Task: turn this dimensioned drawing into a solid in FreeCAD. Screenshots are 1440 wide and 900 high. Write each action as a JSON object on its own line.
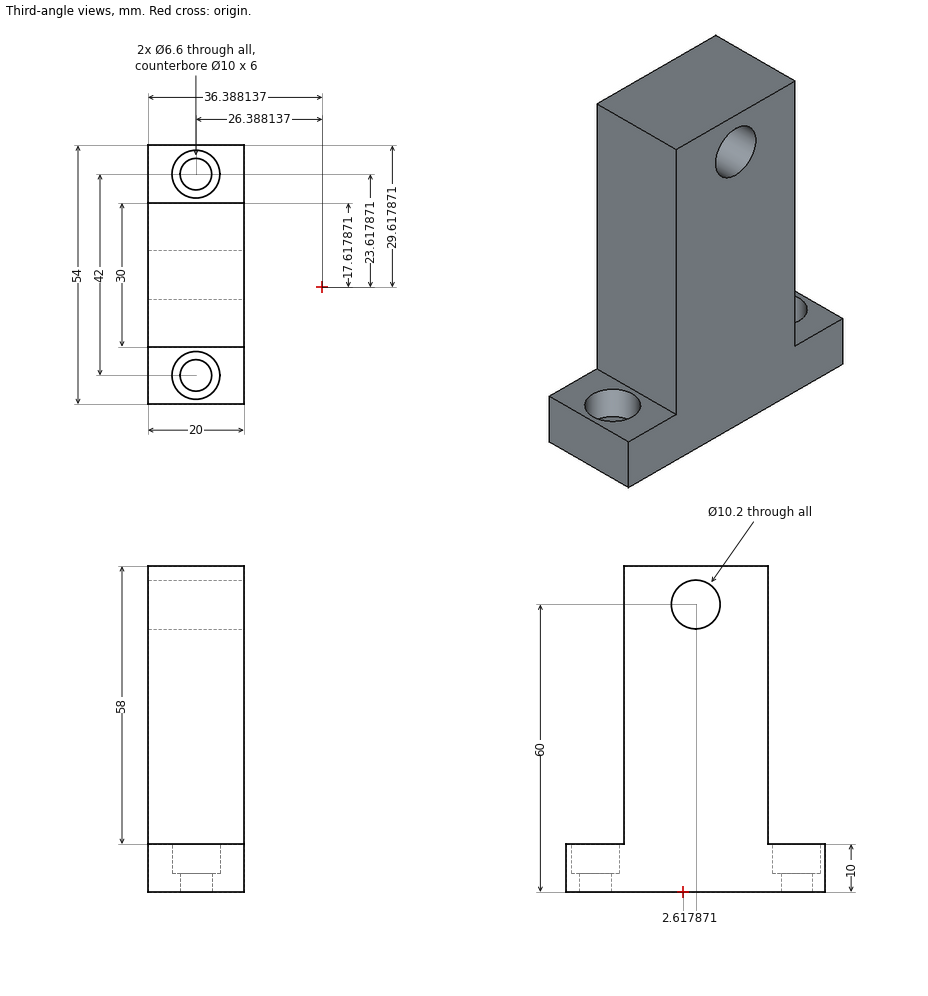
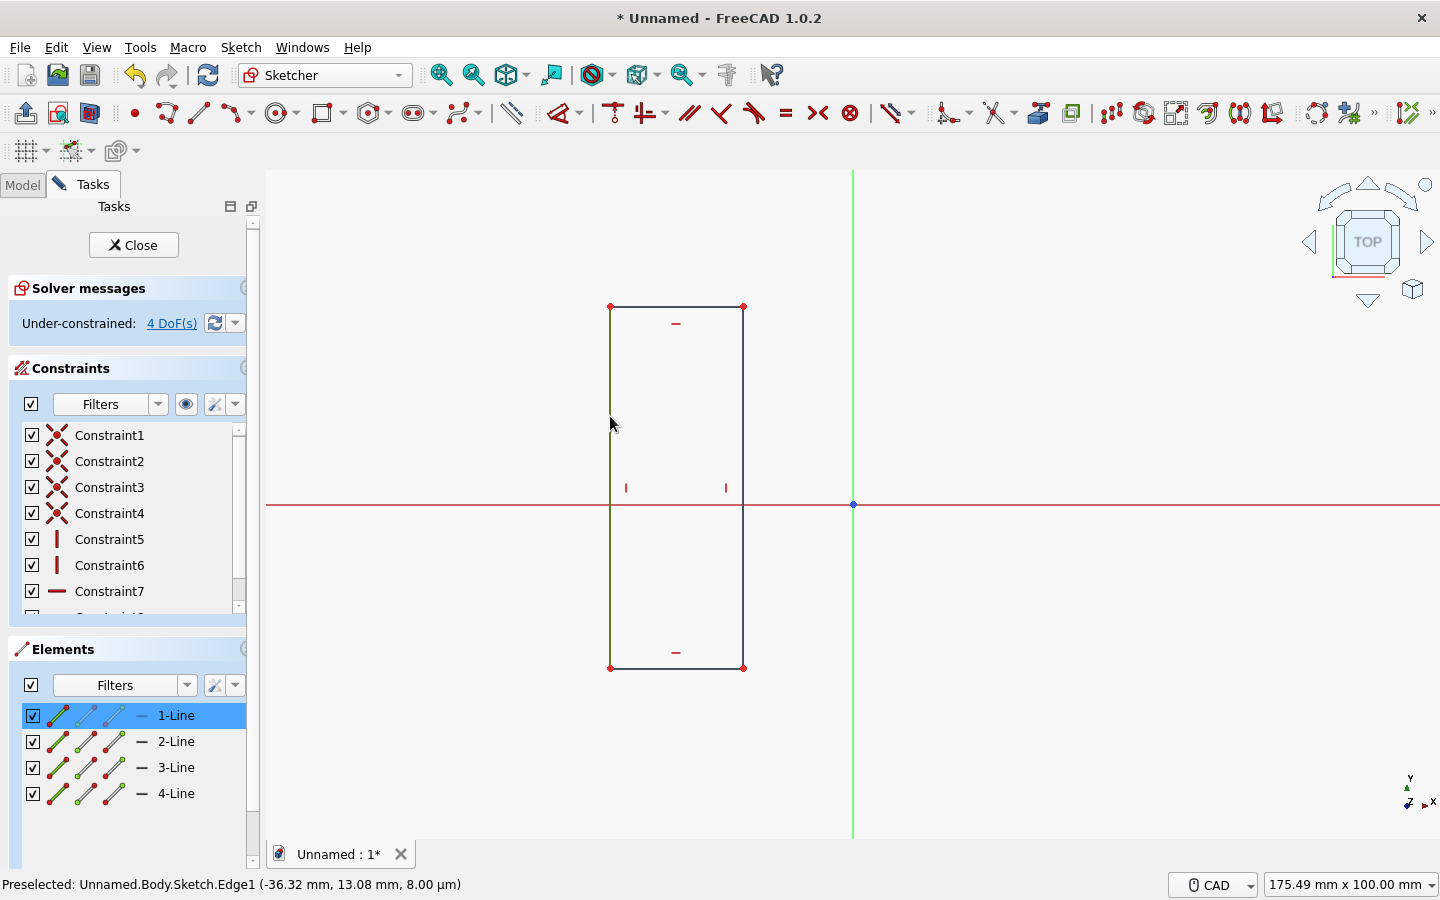
{"action": "left_click", "coordinate": [582, 114]}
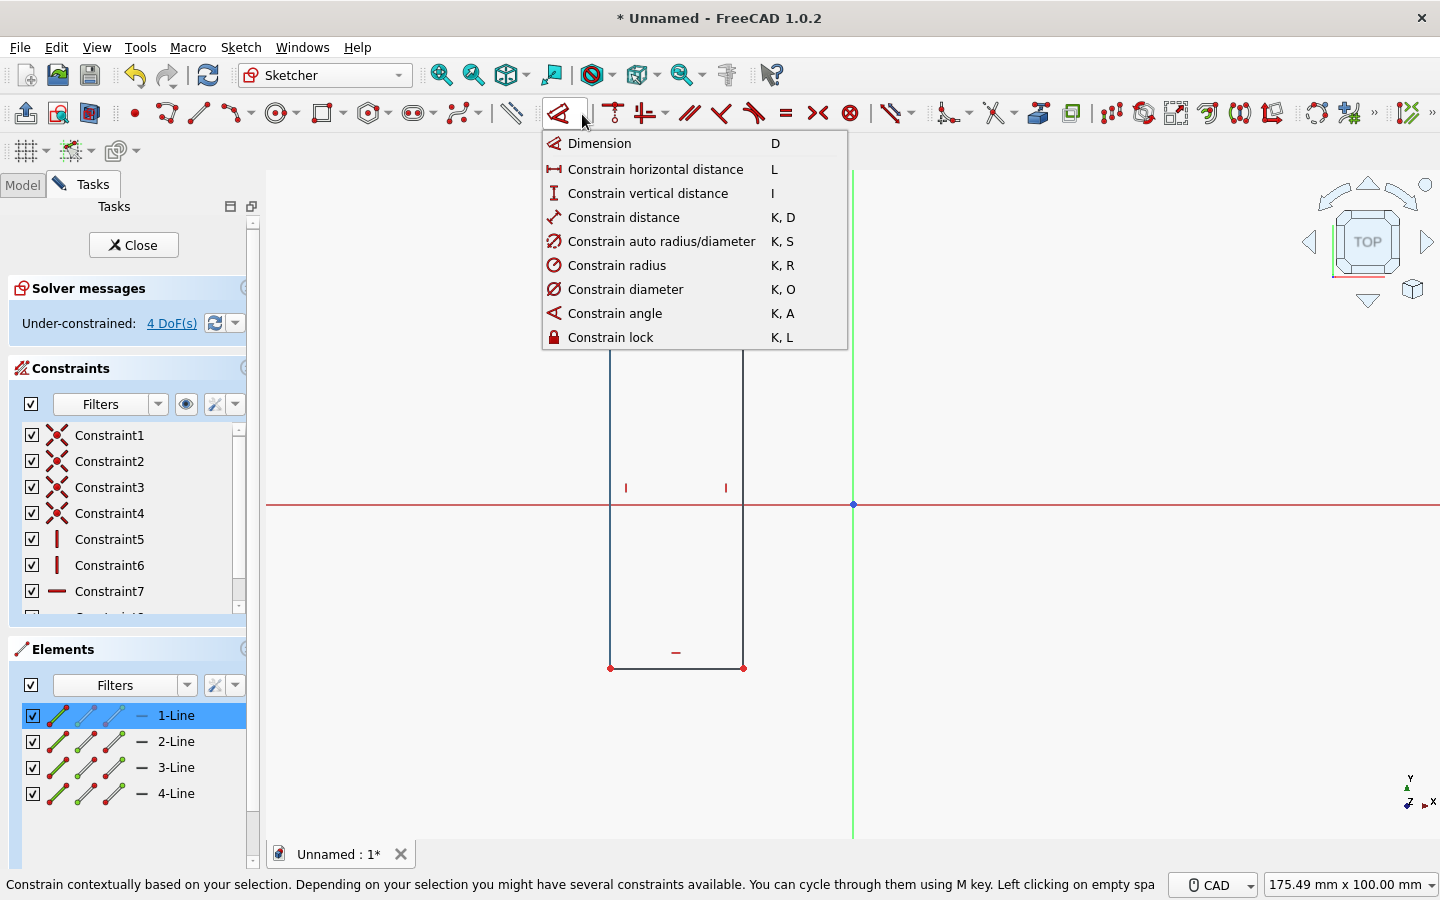
{"action": "left_click", "coordinate": [695, 193]}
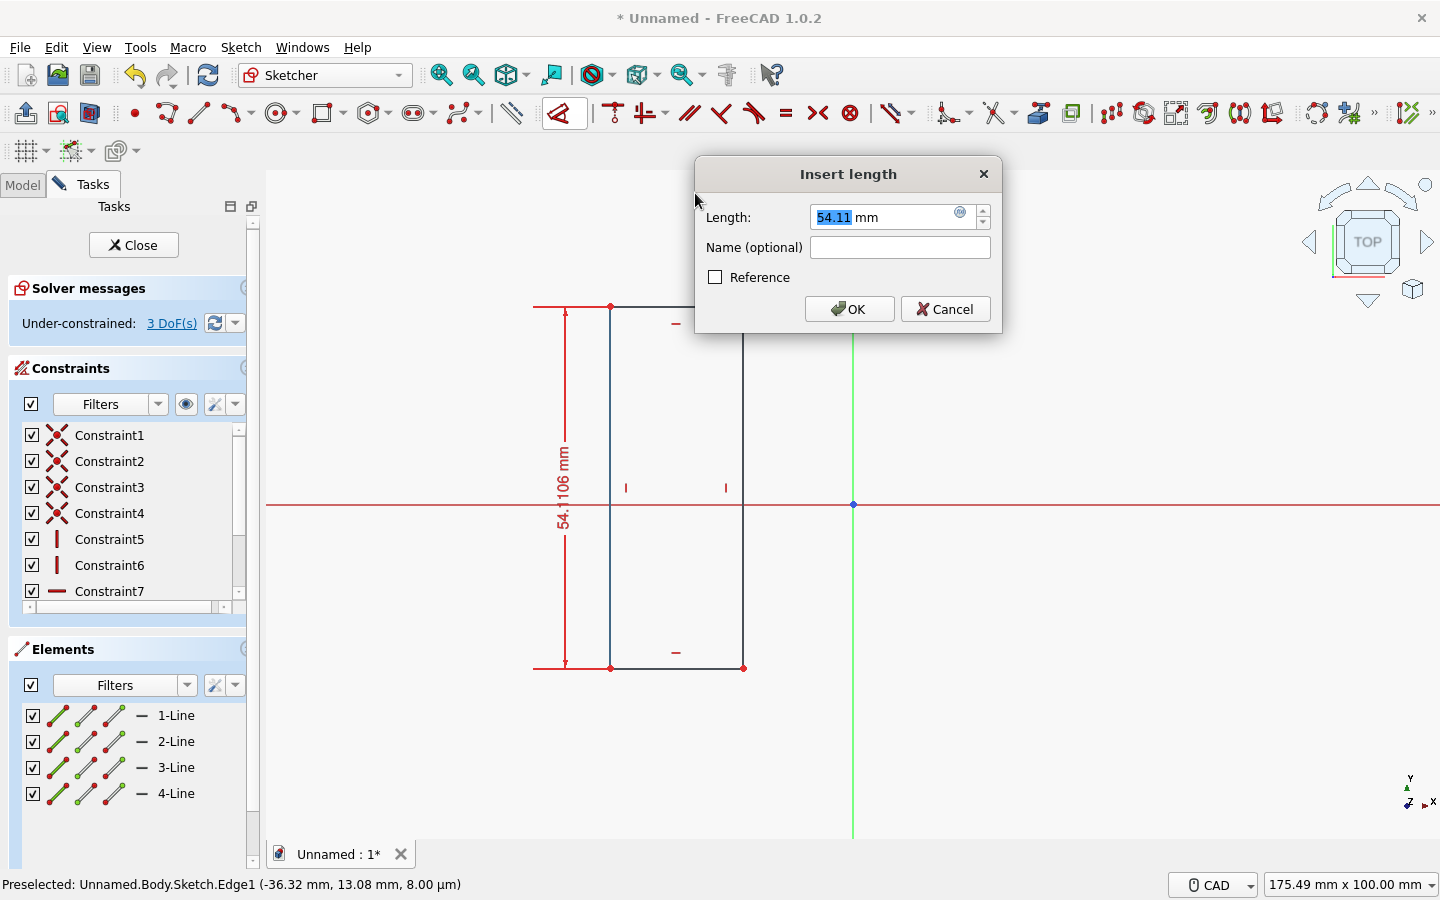
{"action": "type", "text": "54"}
{"action": "key", "text": "Return"}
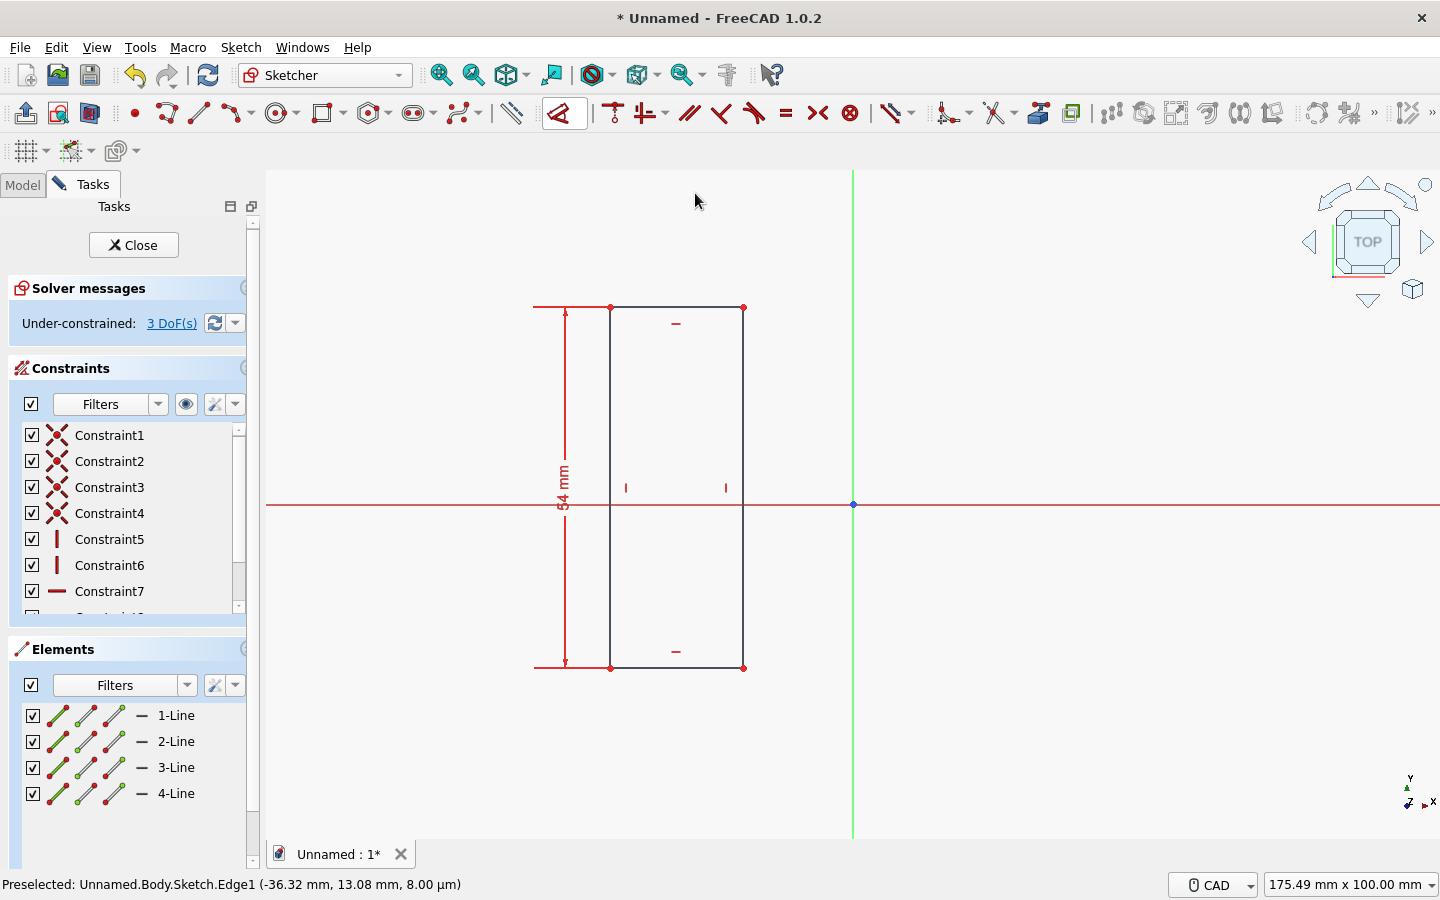
{"action": "left_click", "coordinate": [650, 668]}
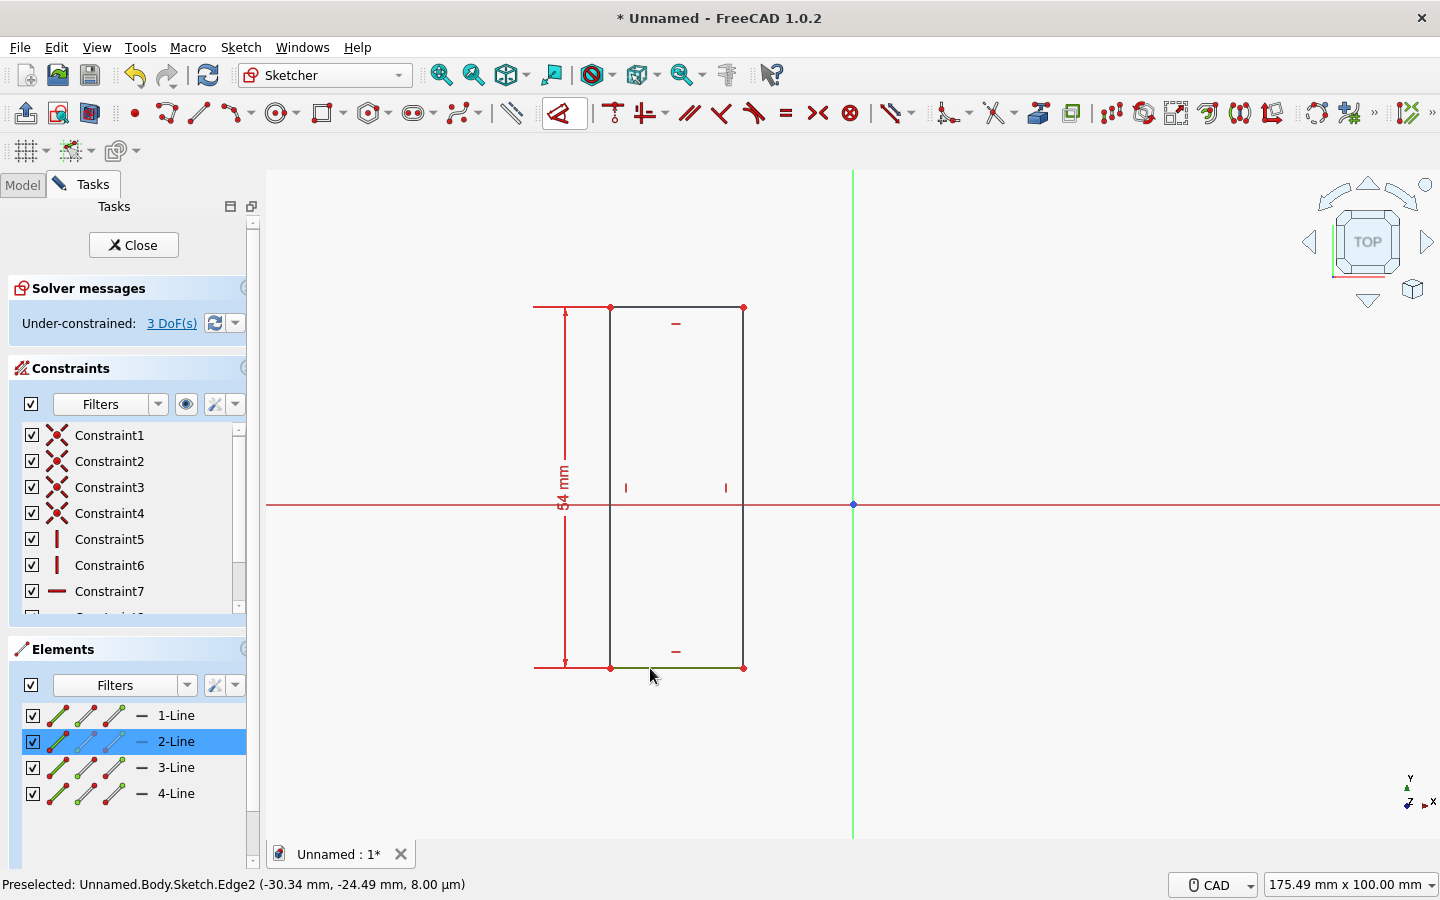
{"action": "left_click", "coordinate": [582, 114]}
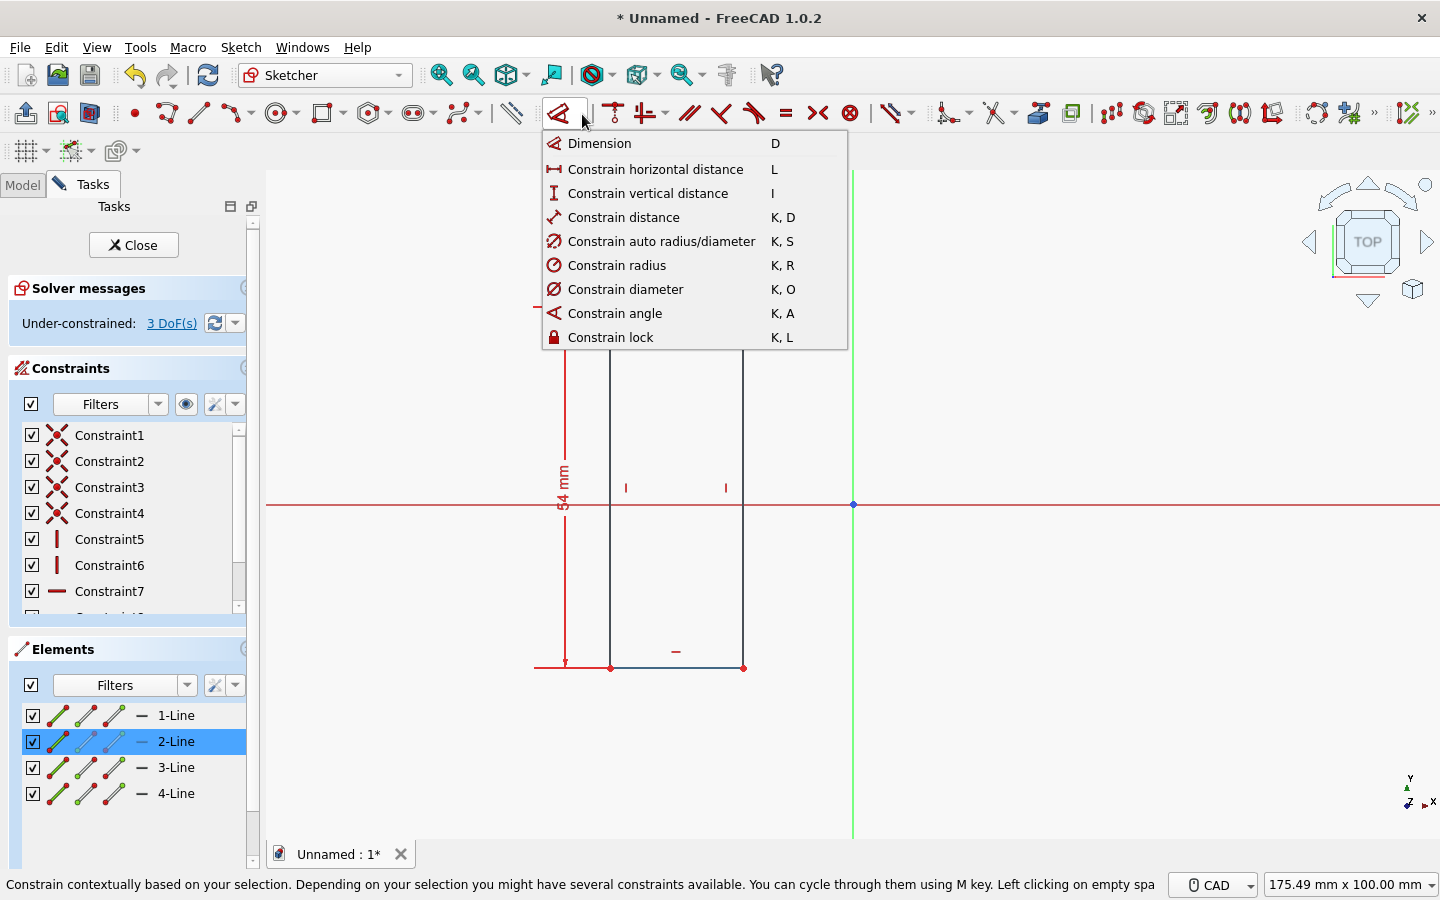
{"action": "left_click", "coordinate": [695, 169]}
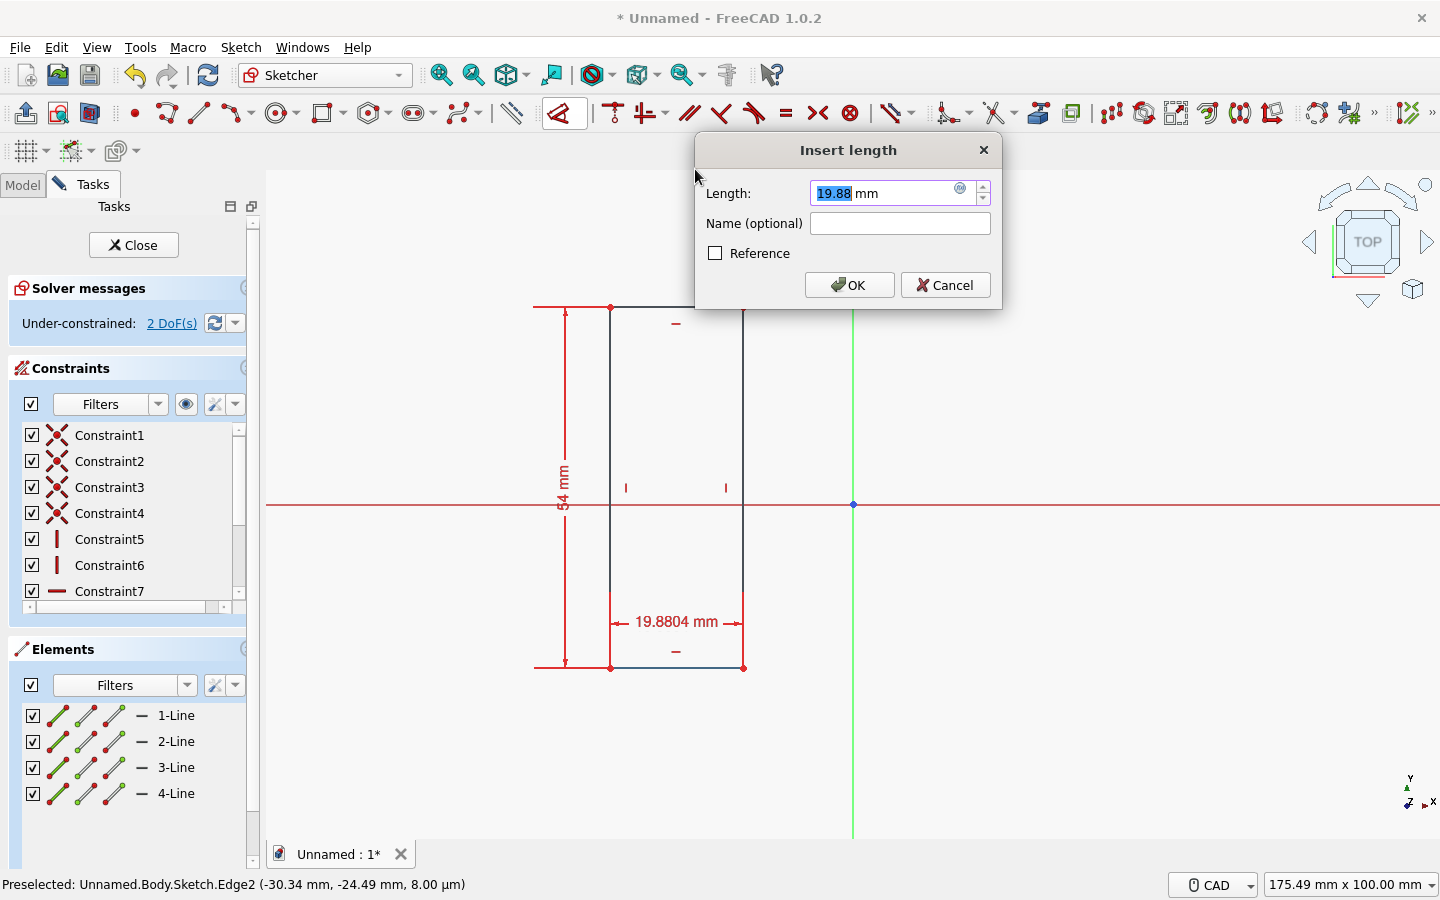
{"action": "type", "text": "20"}
{"action": "key", "text": "Return"}